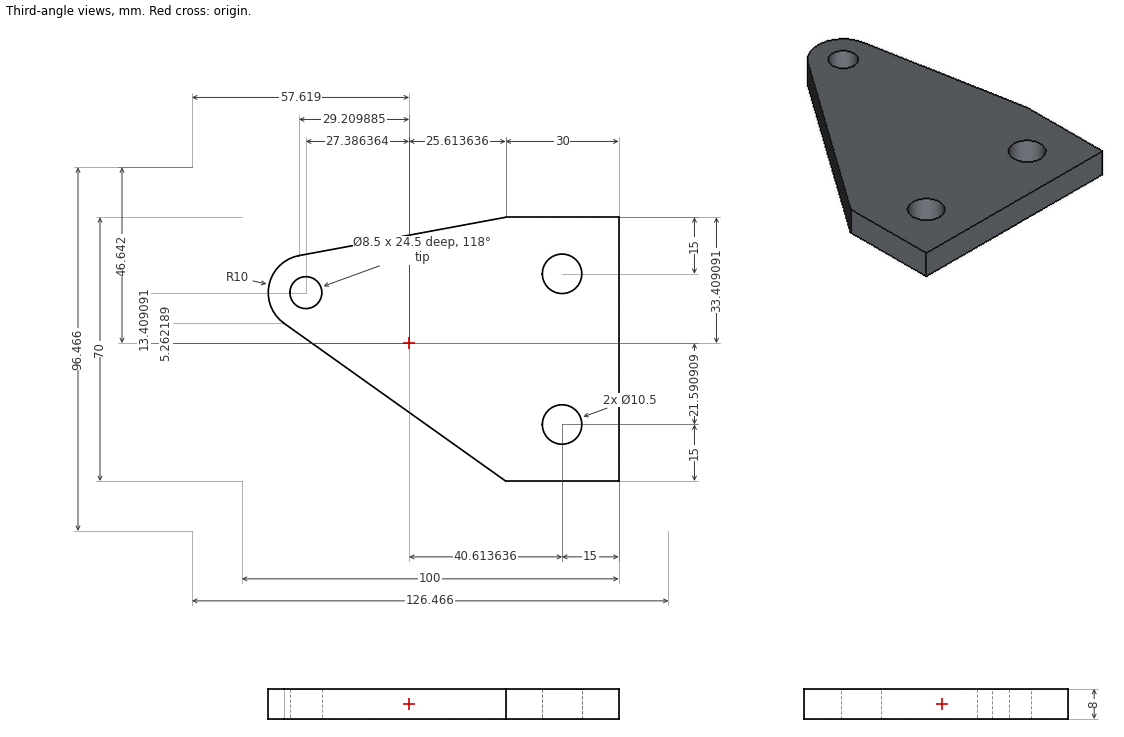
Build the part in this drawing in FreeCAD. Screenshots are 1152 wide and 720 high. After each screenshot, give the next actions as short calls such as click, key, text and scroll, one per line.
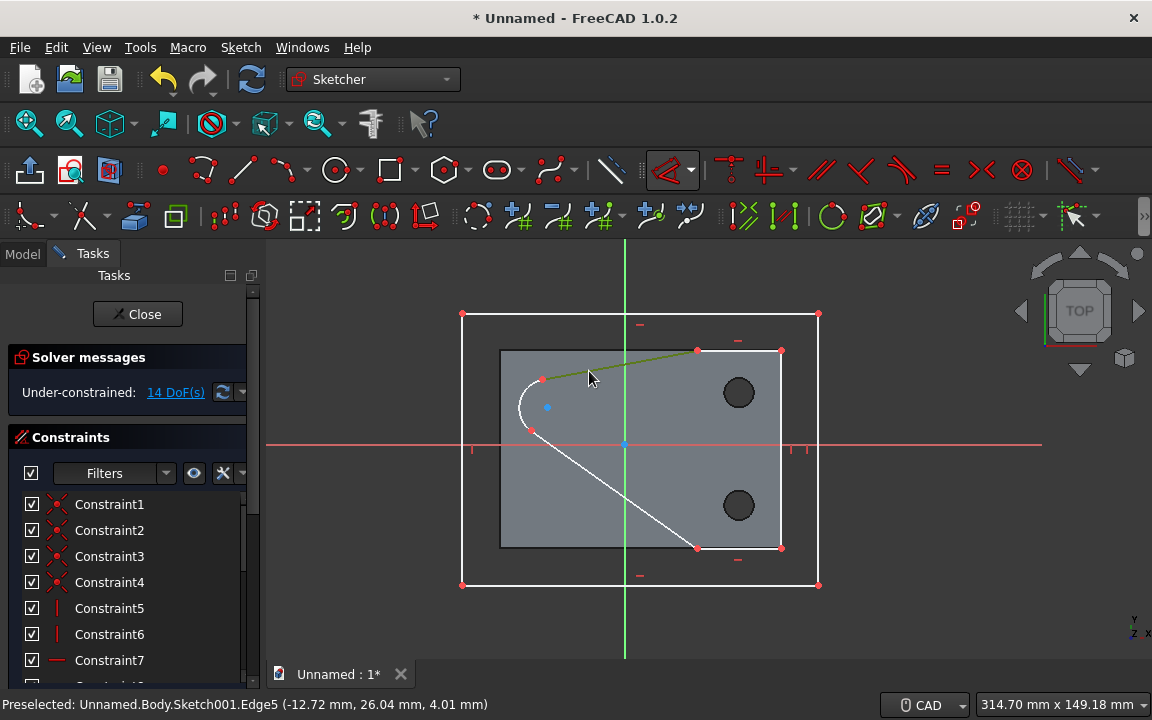
click(526, 390)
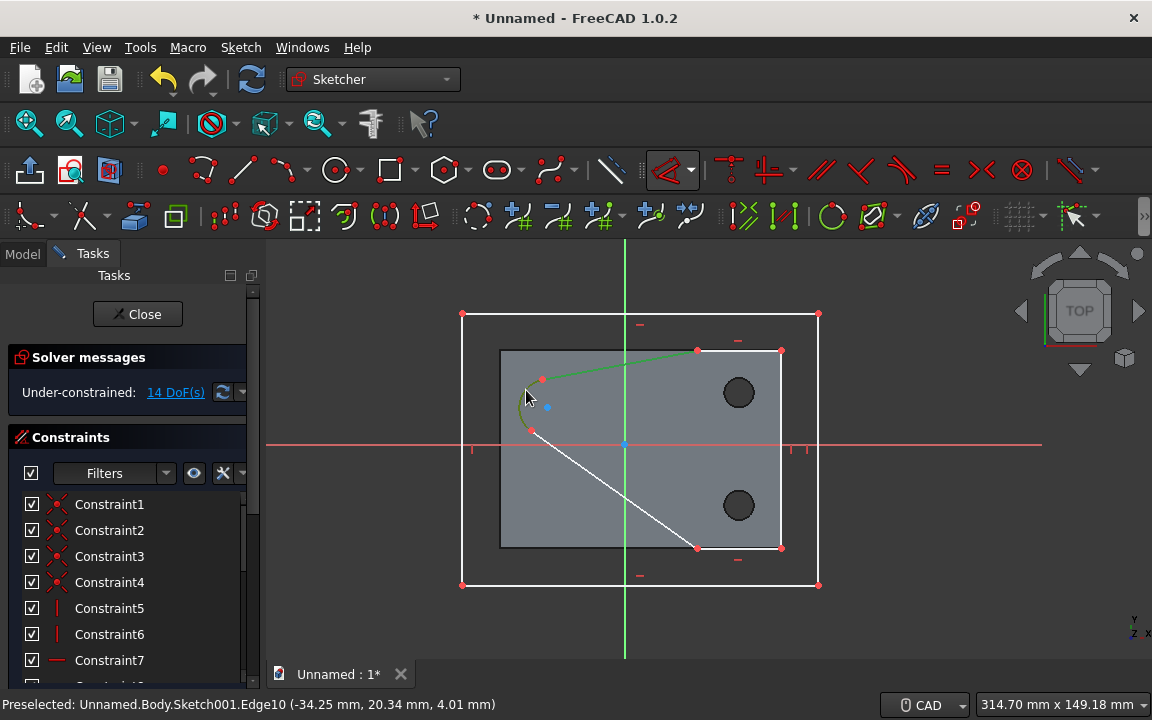
click(902, 170)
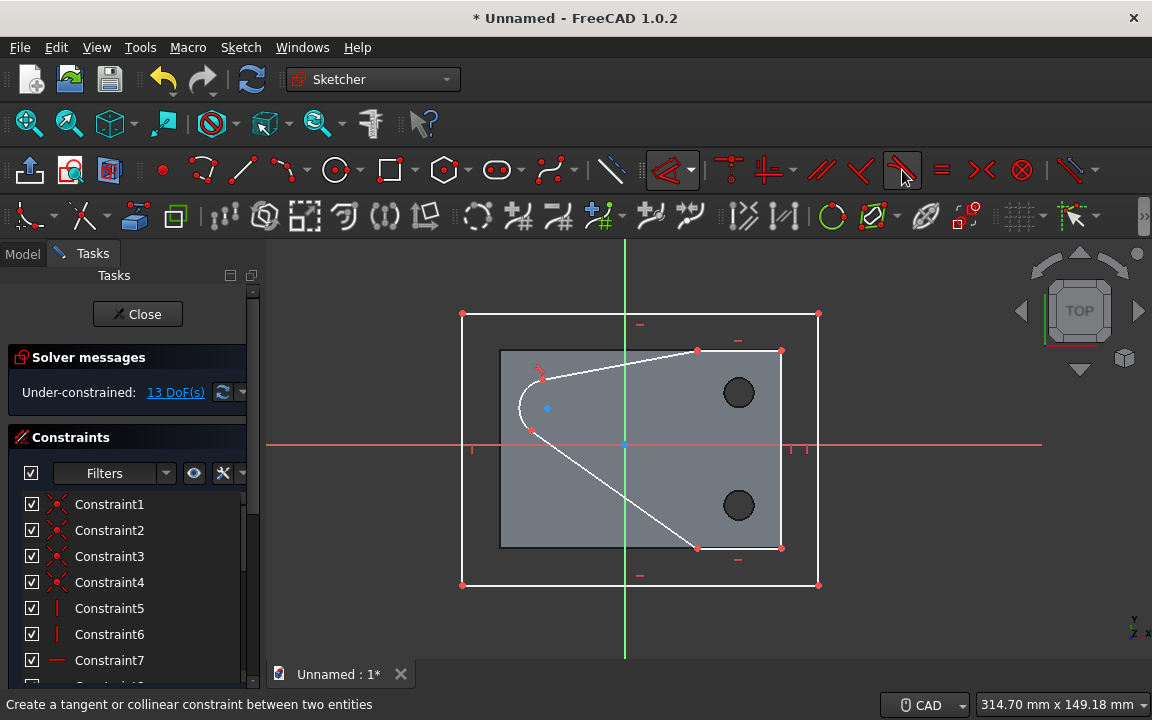
click(647, 514)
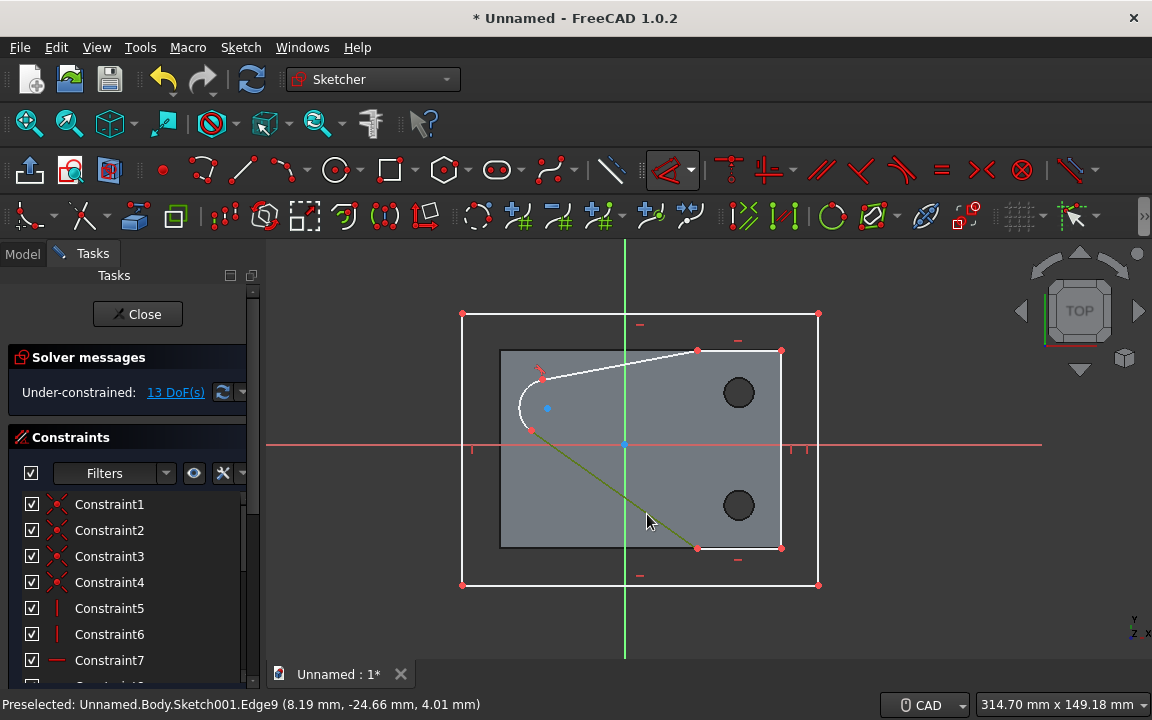
click(526, 390)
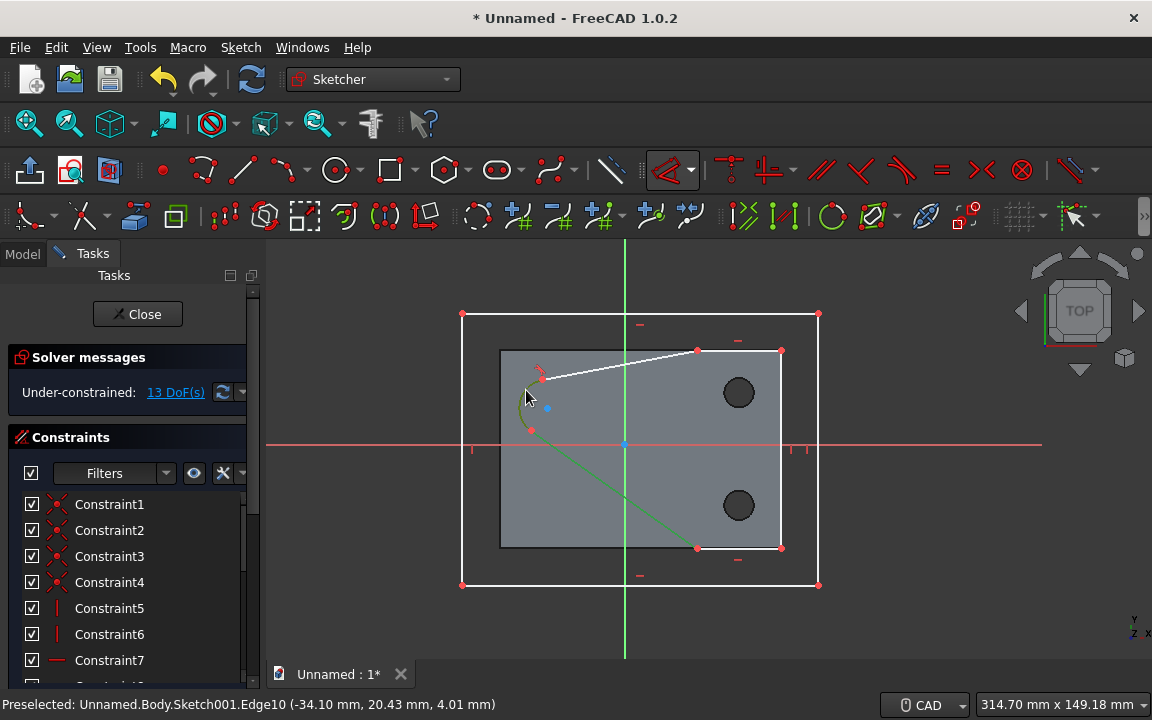
click(902, 170)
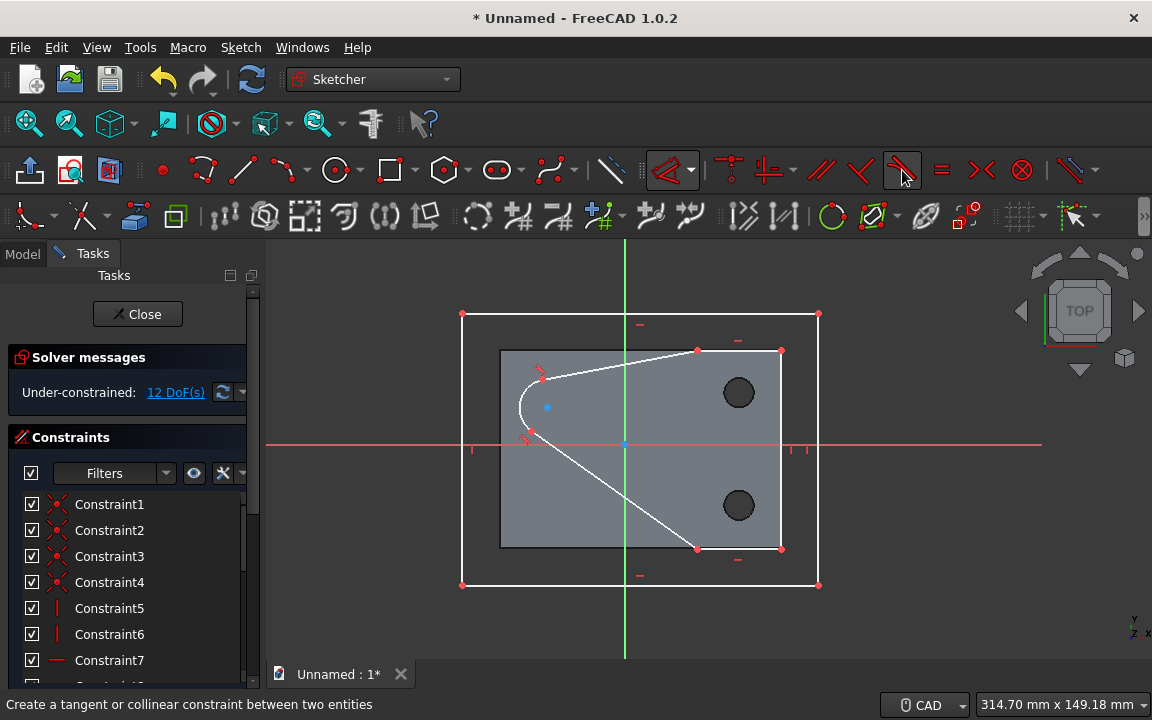
click(666, 170)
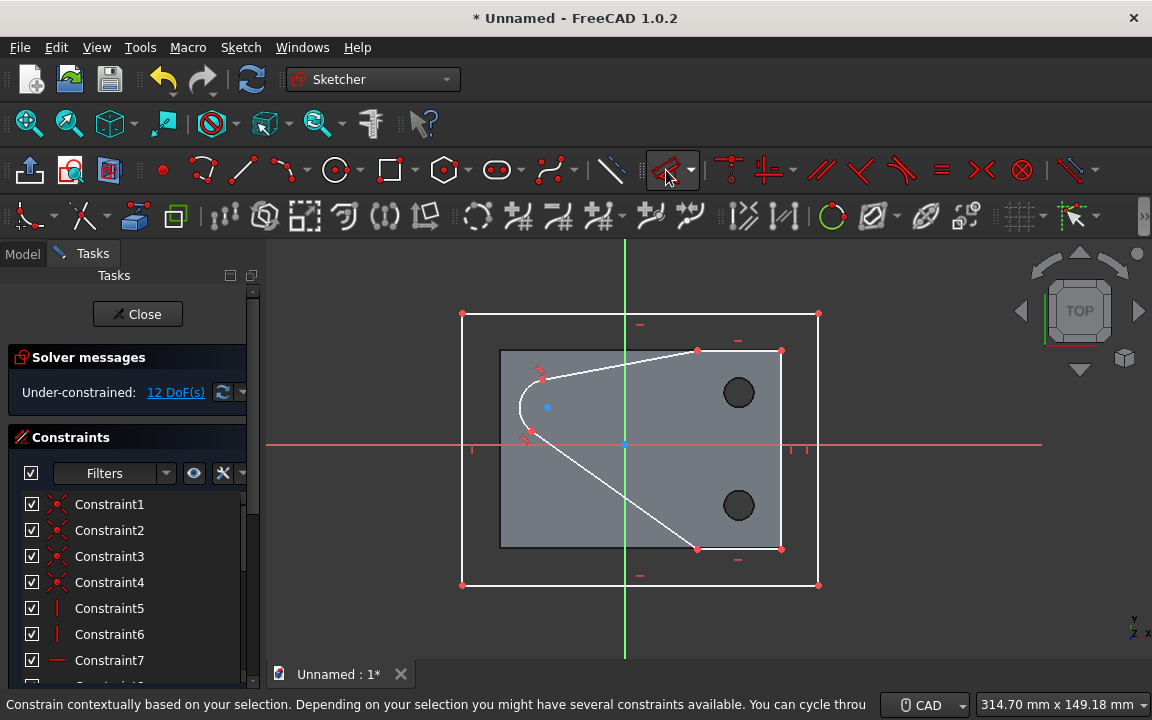
scroll(526, 390, up, 2)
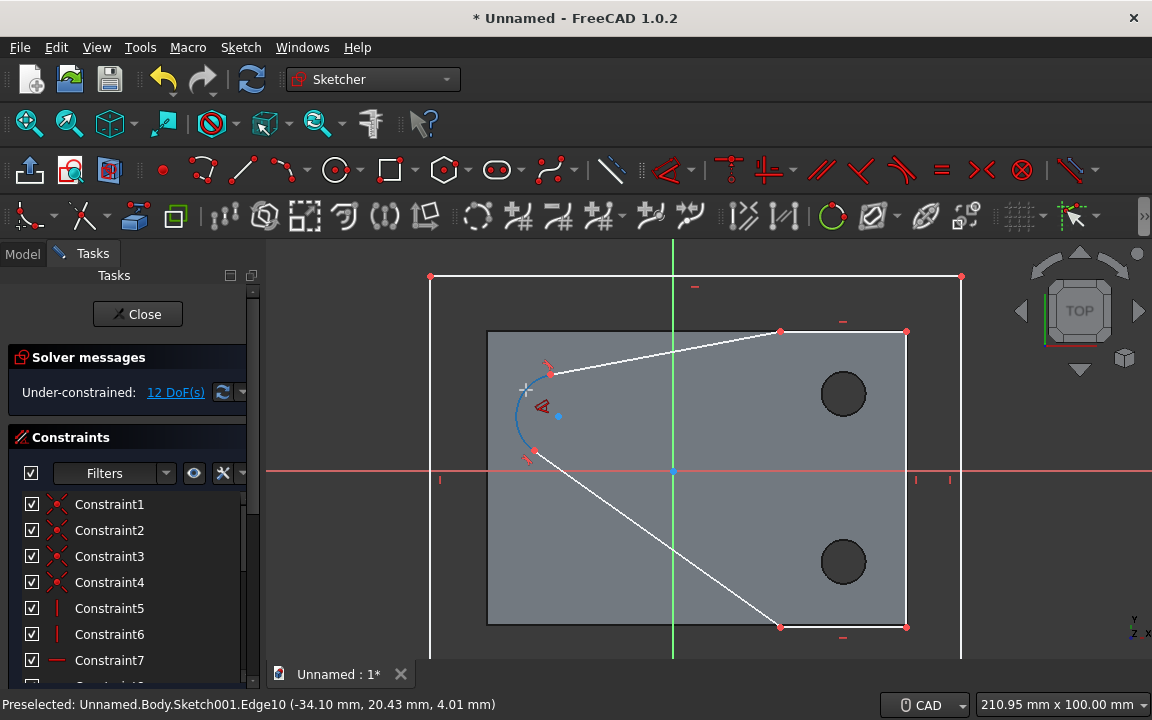
click(526, 390)
click(501, 370)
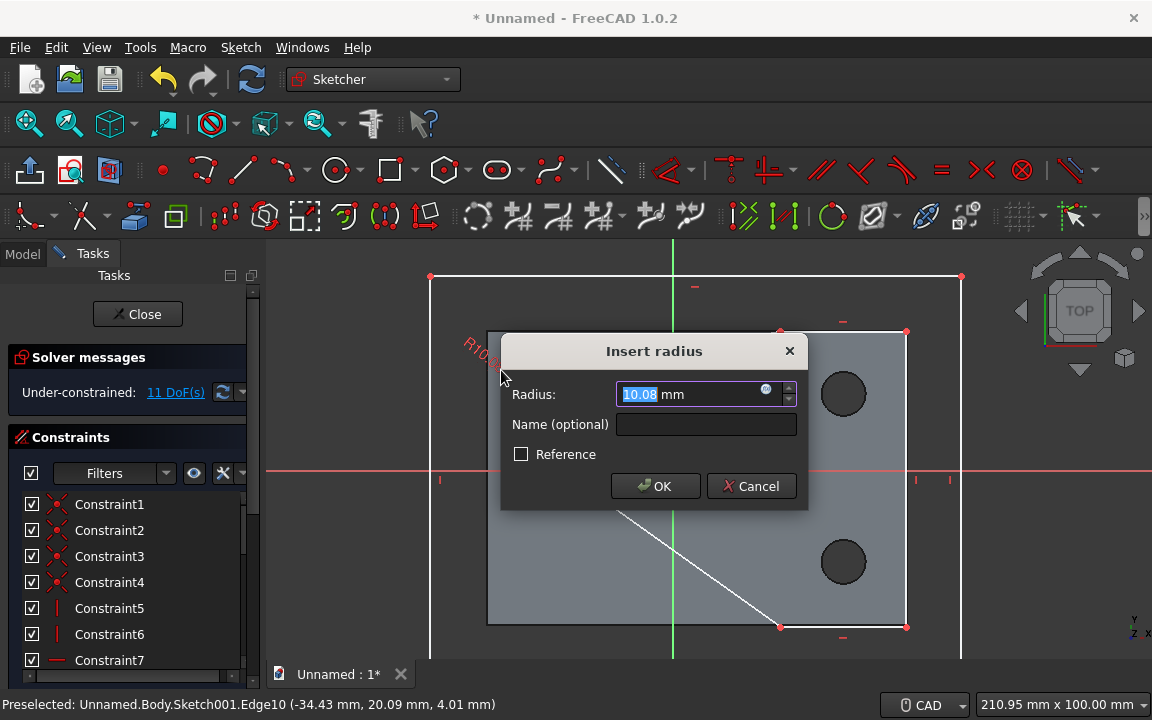
text(10)
key(Return)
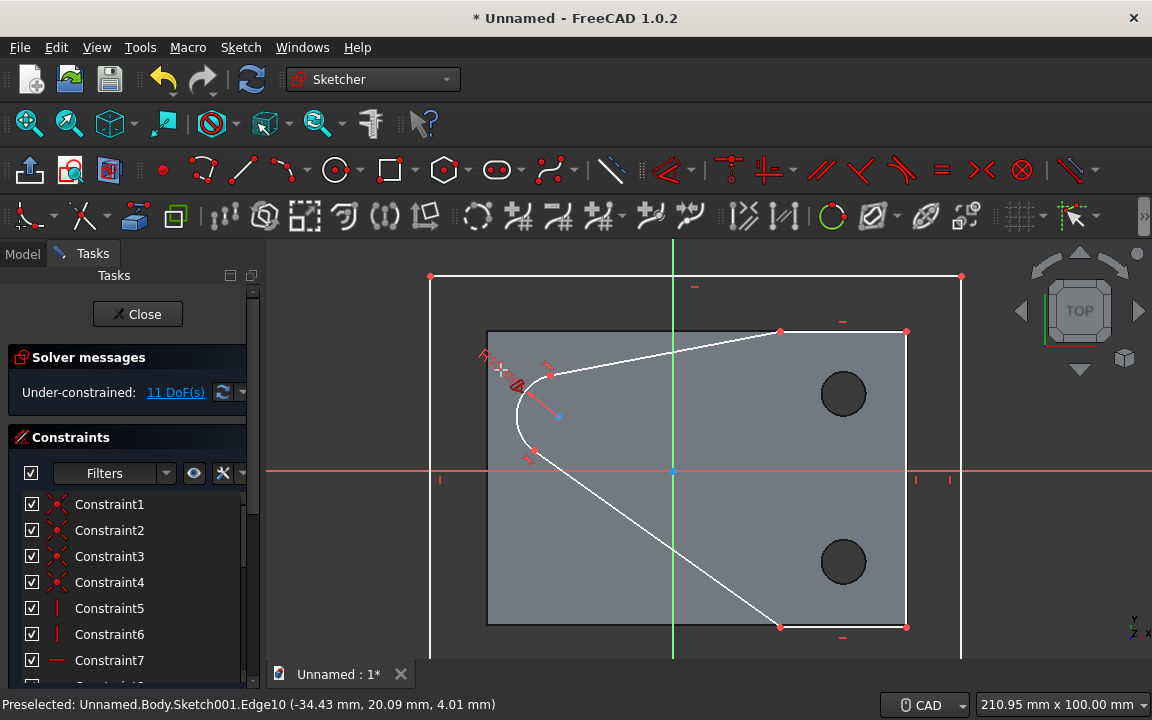
click(819, 332)
click(844, 298)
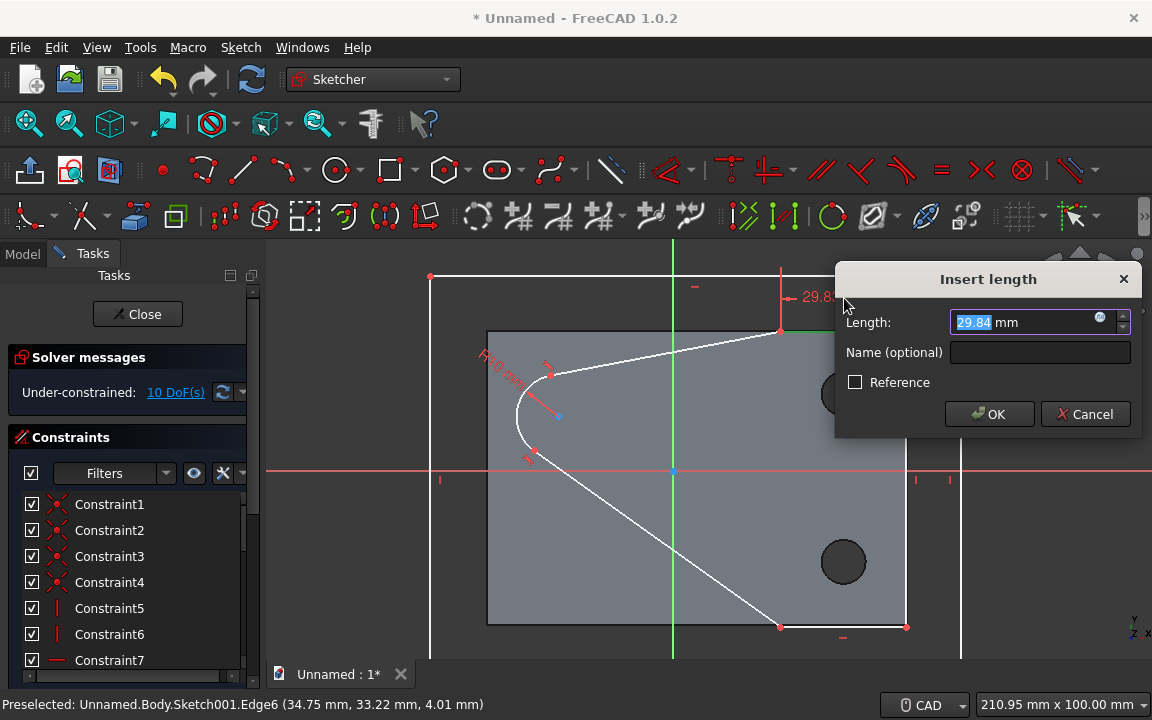
text(30)
key(Return)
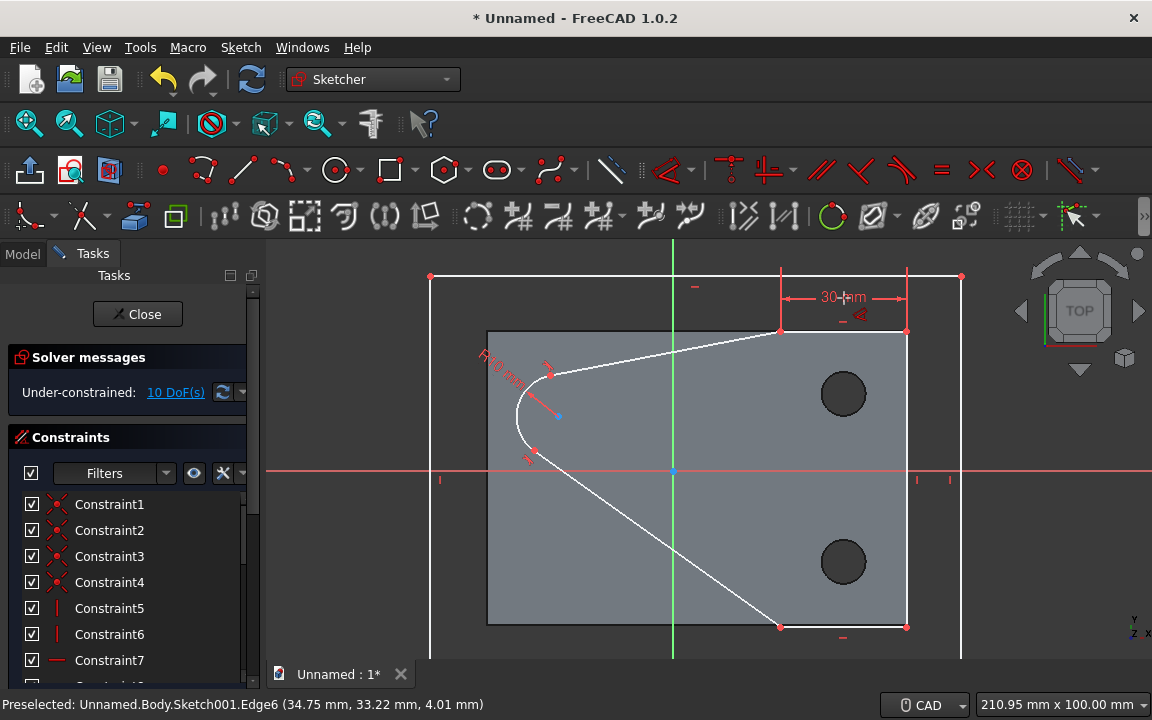
click(907, 420)
click(941, 411)